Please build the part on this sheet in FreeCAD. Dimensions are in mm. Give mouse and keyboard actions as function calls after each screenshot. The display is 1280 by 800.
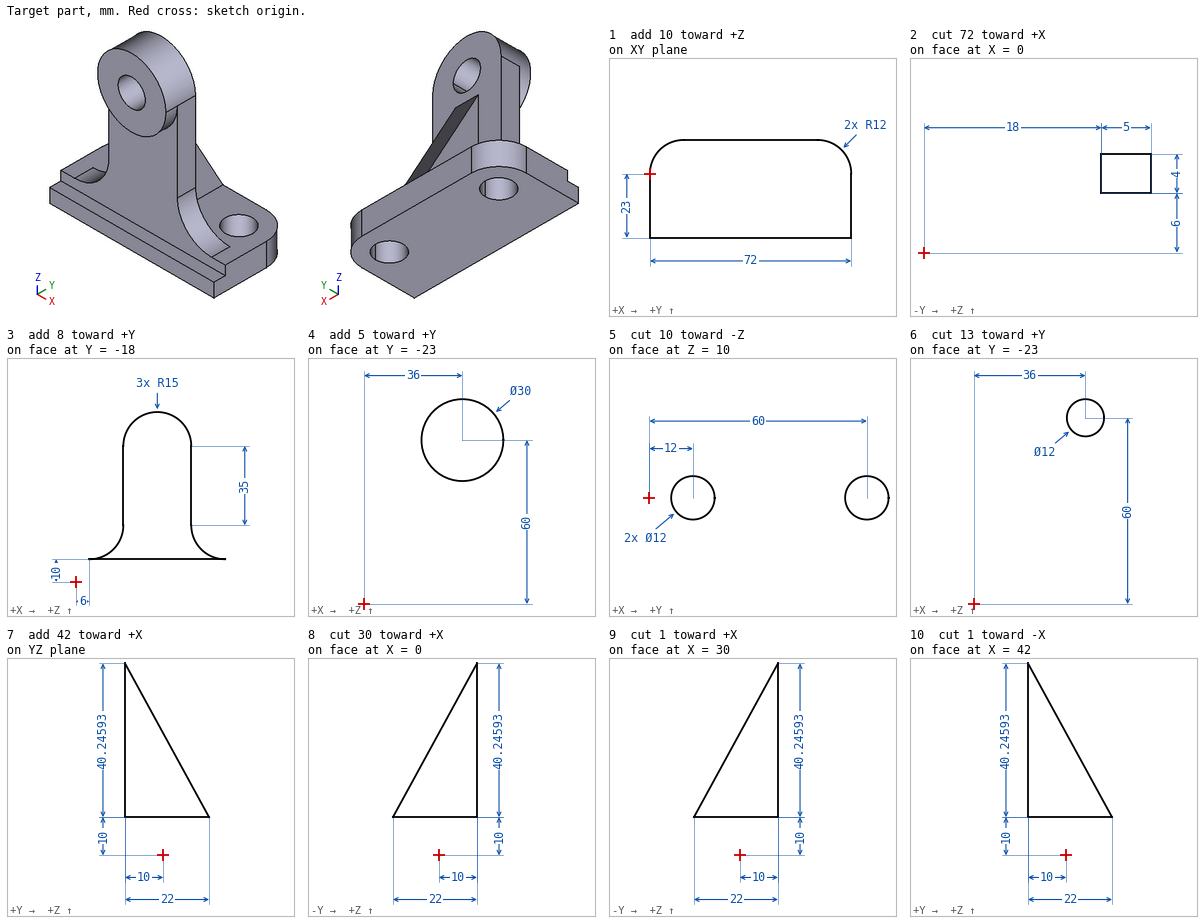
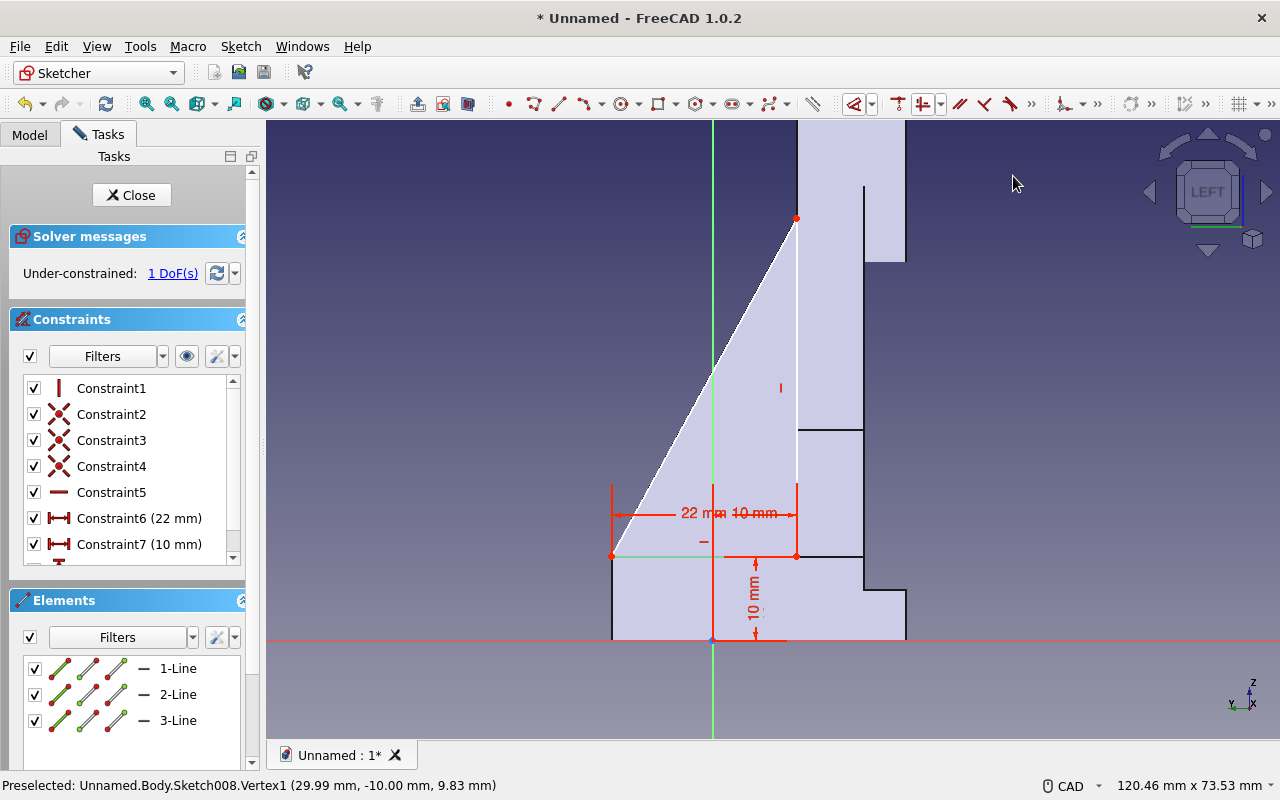
click(797, 455)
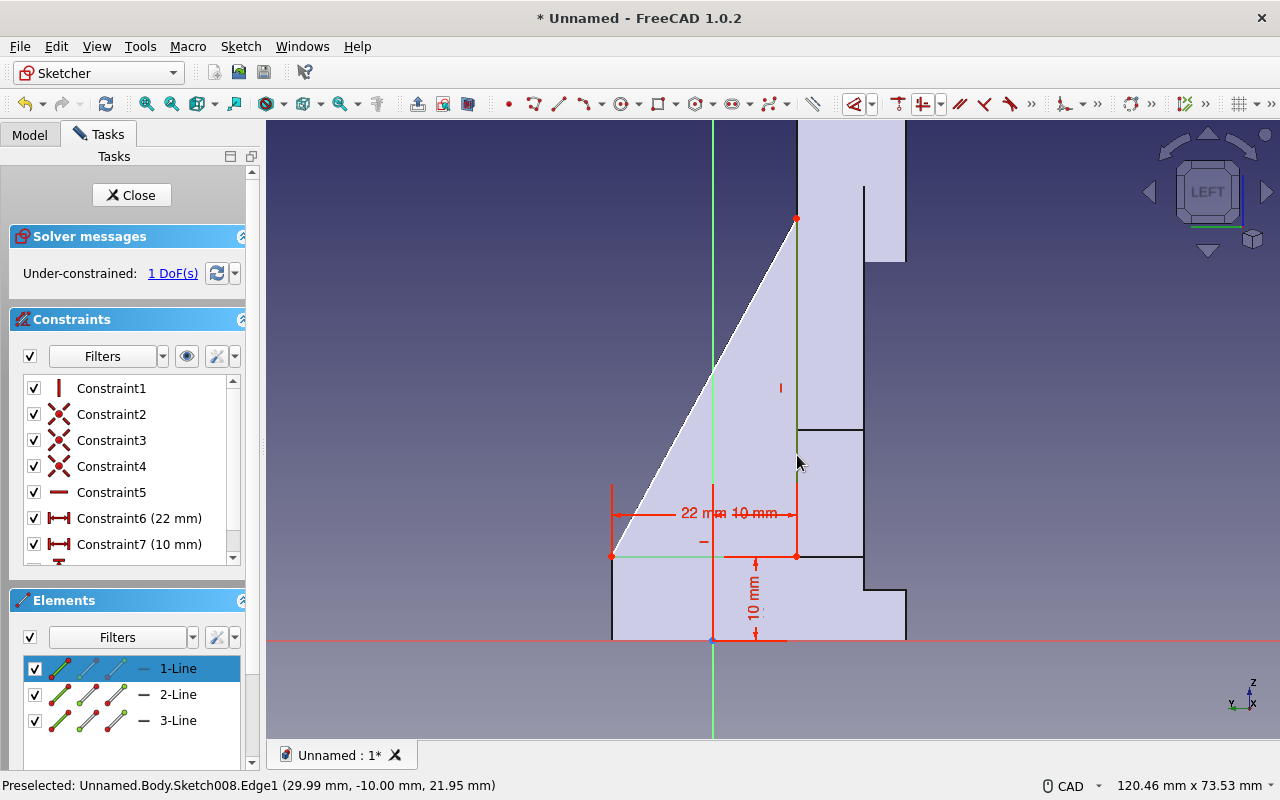
key(i)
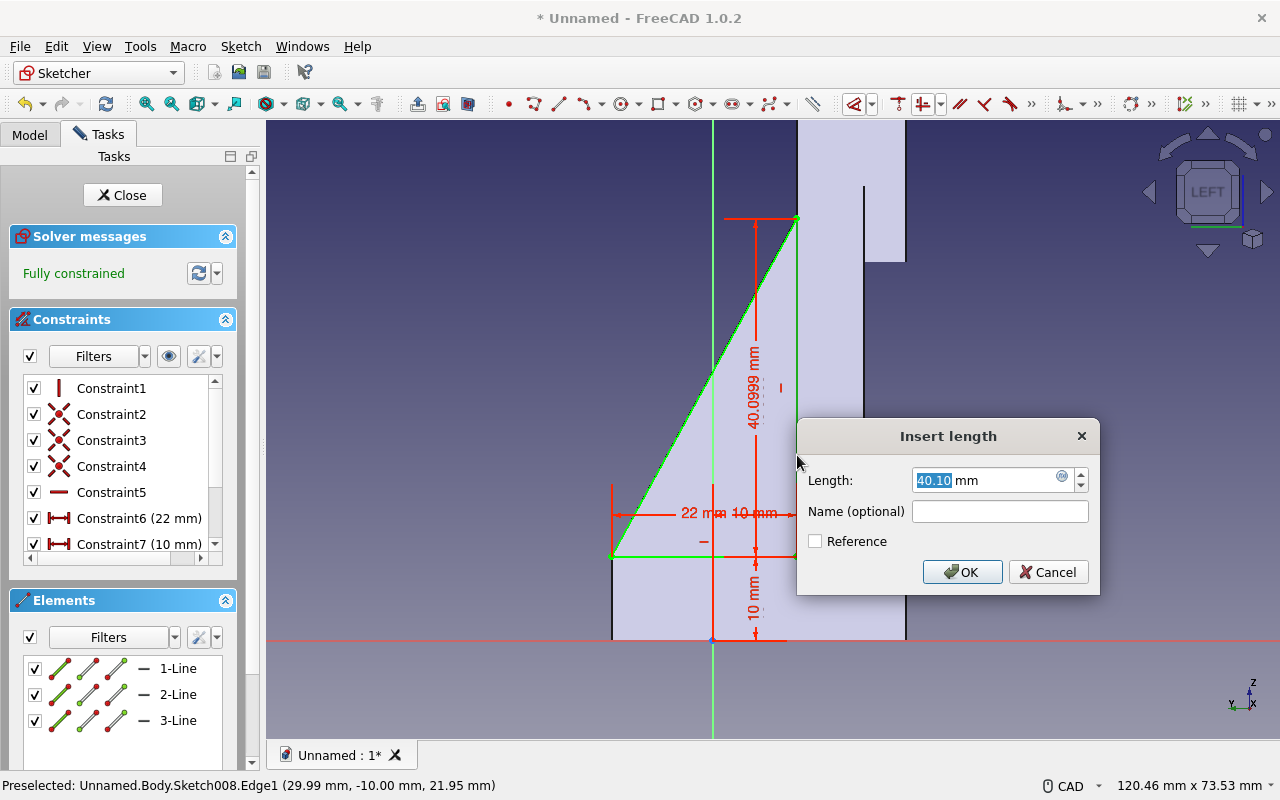
text(40.24593)
key(Return)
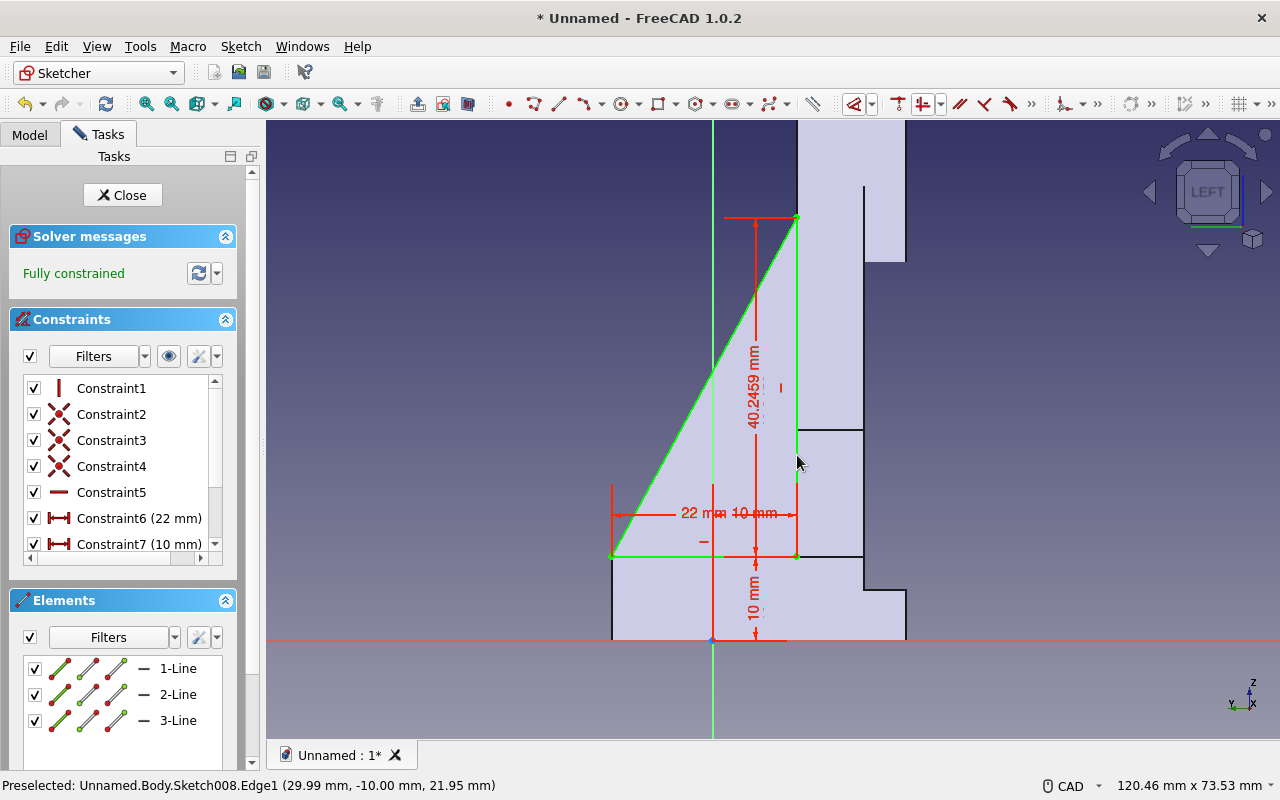
click(123, 195)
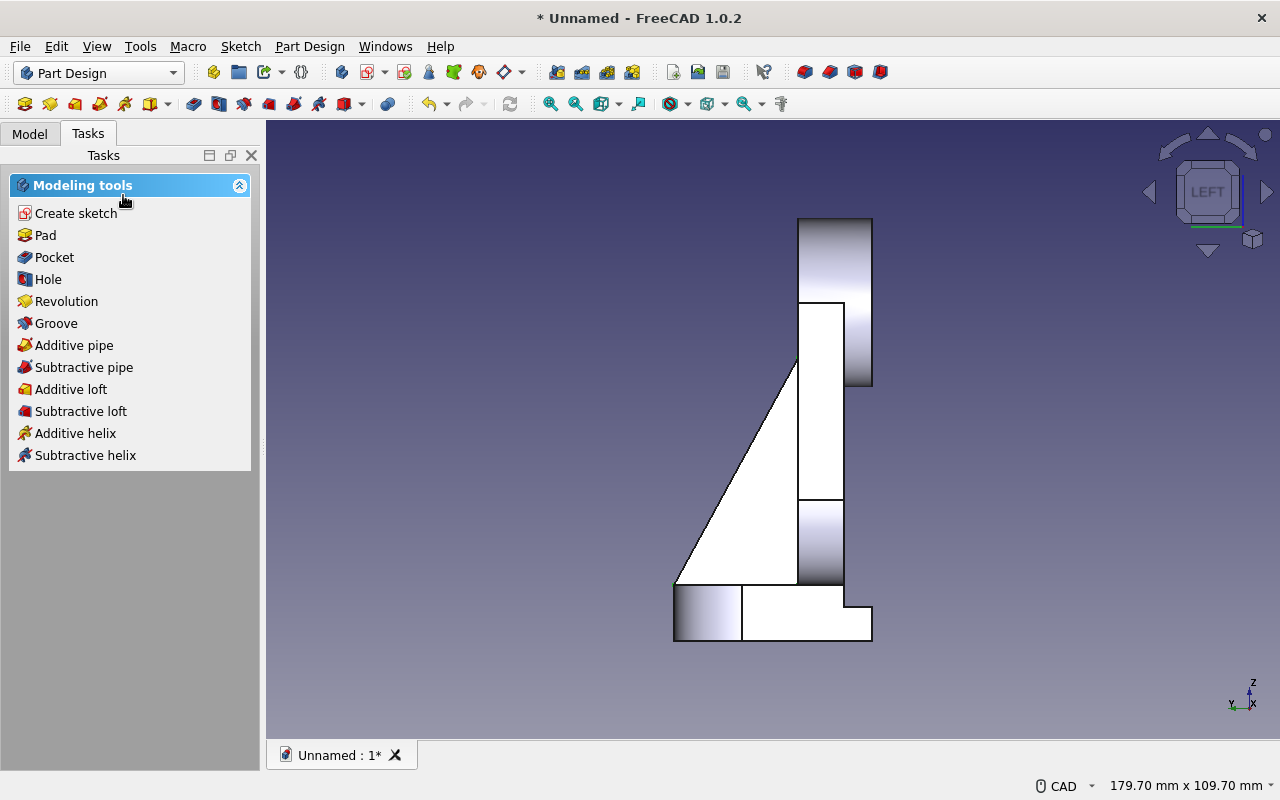
click(194, 104)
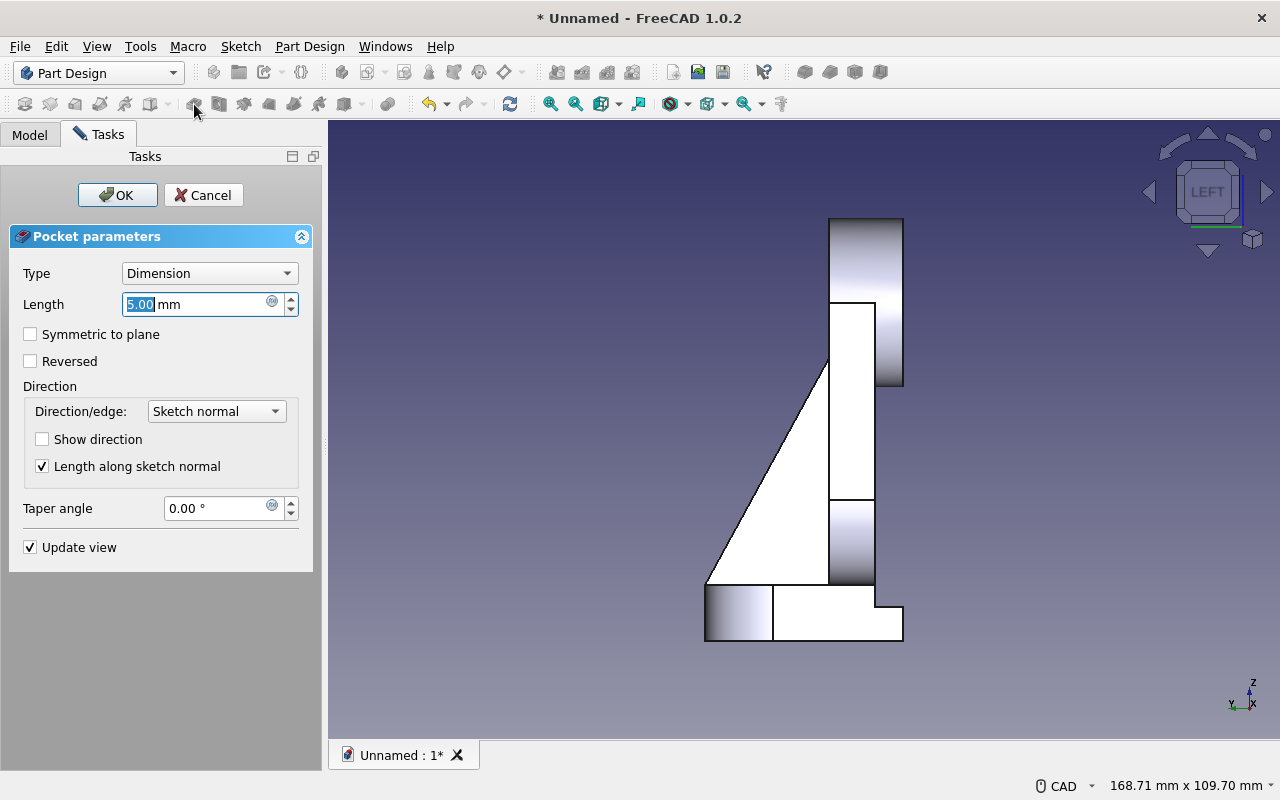
text(1)
key(Tab)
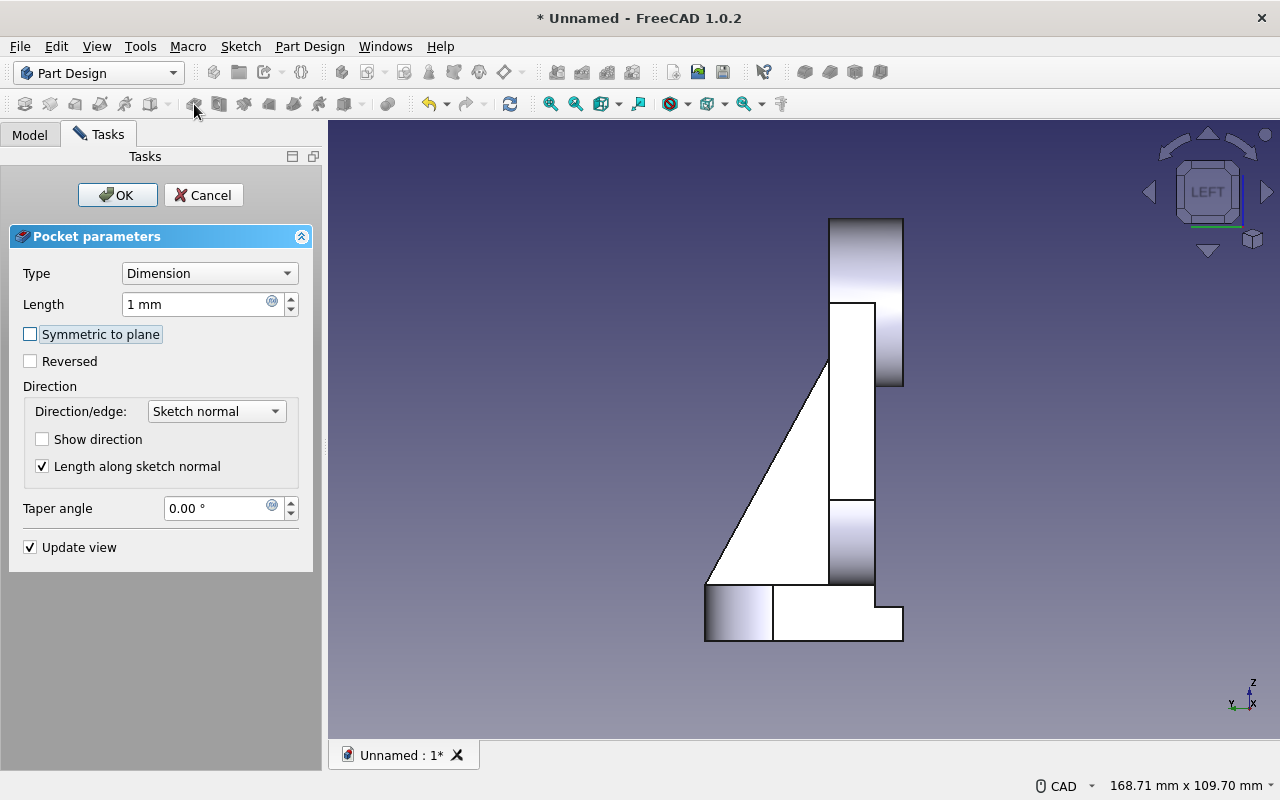
click(118, 195)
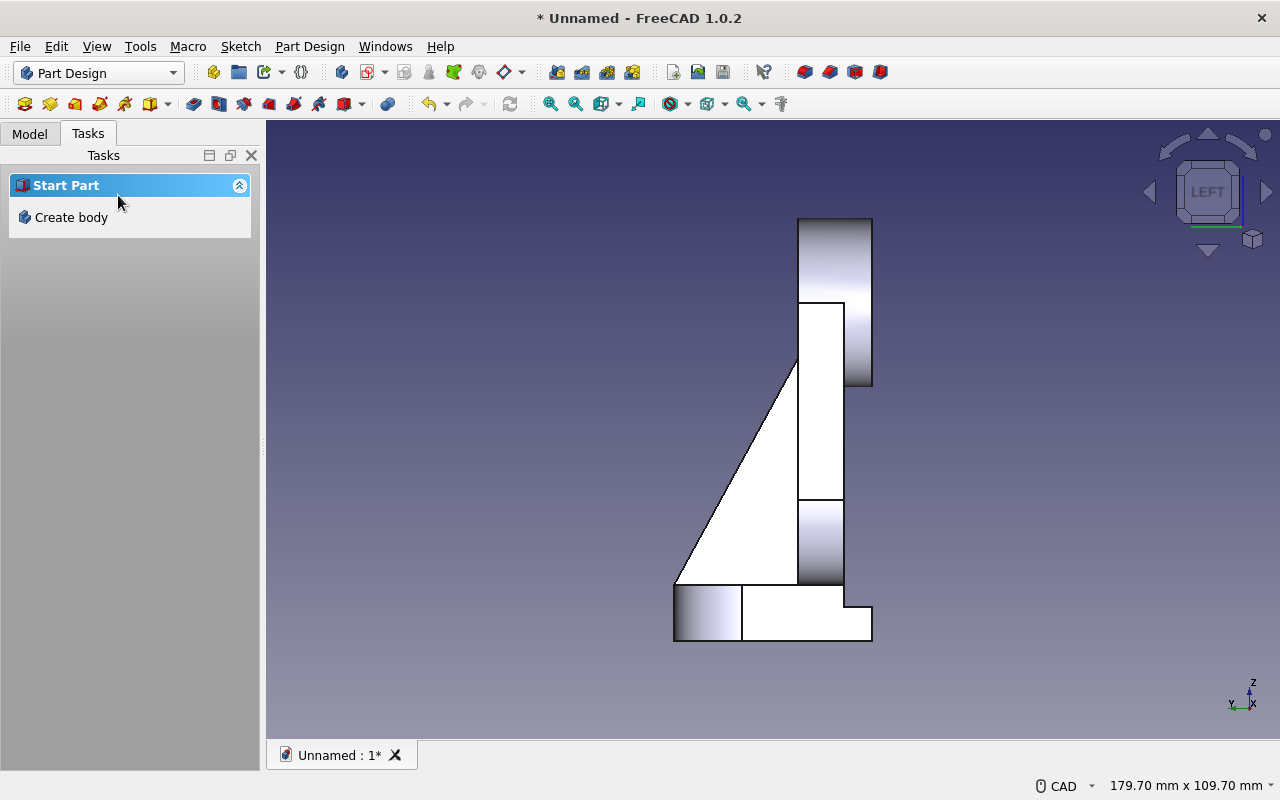
key(0)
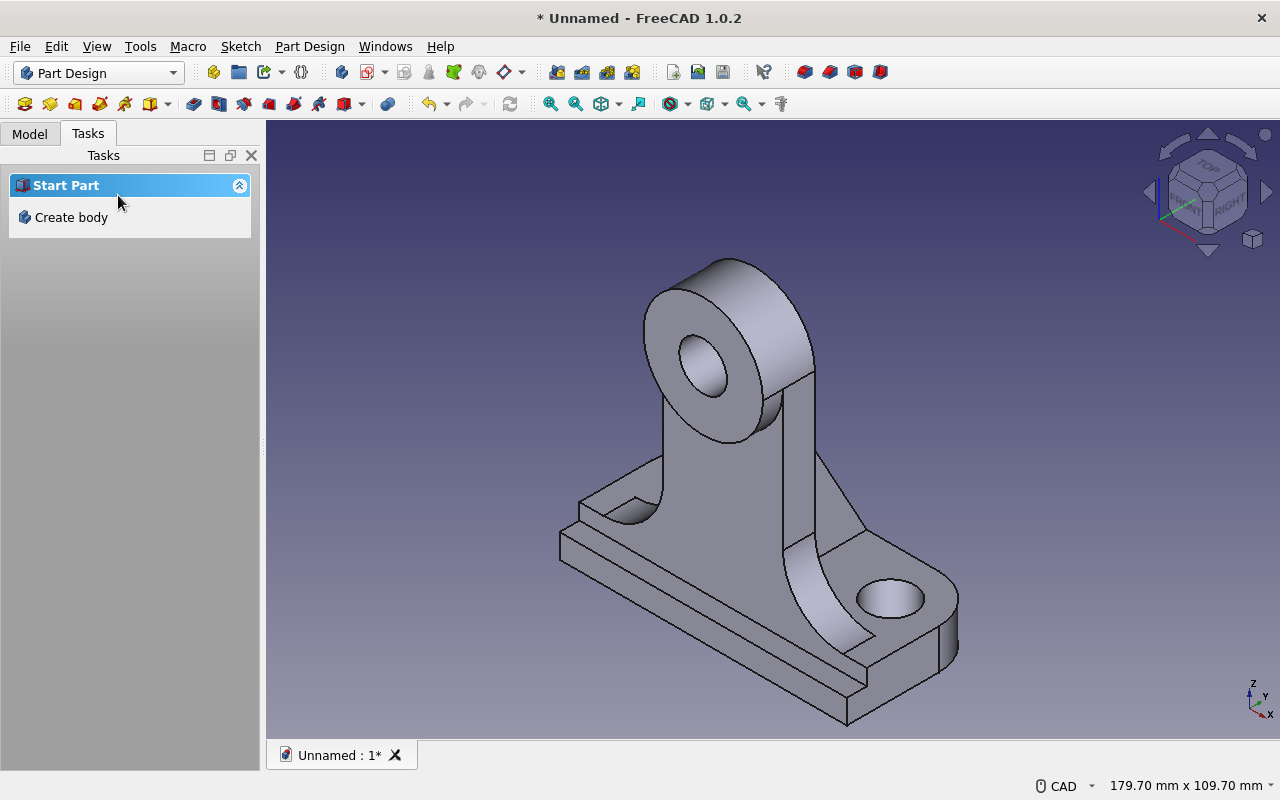
click(823, 514)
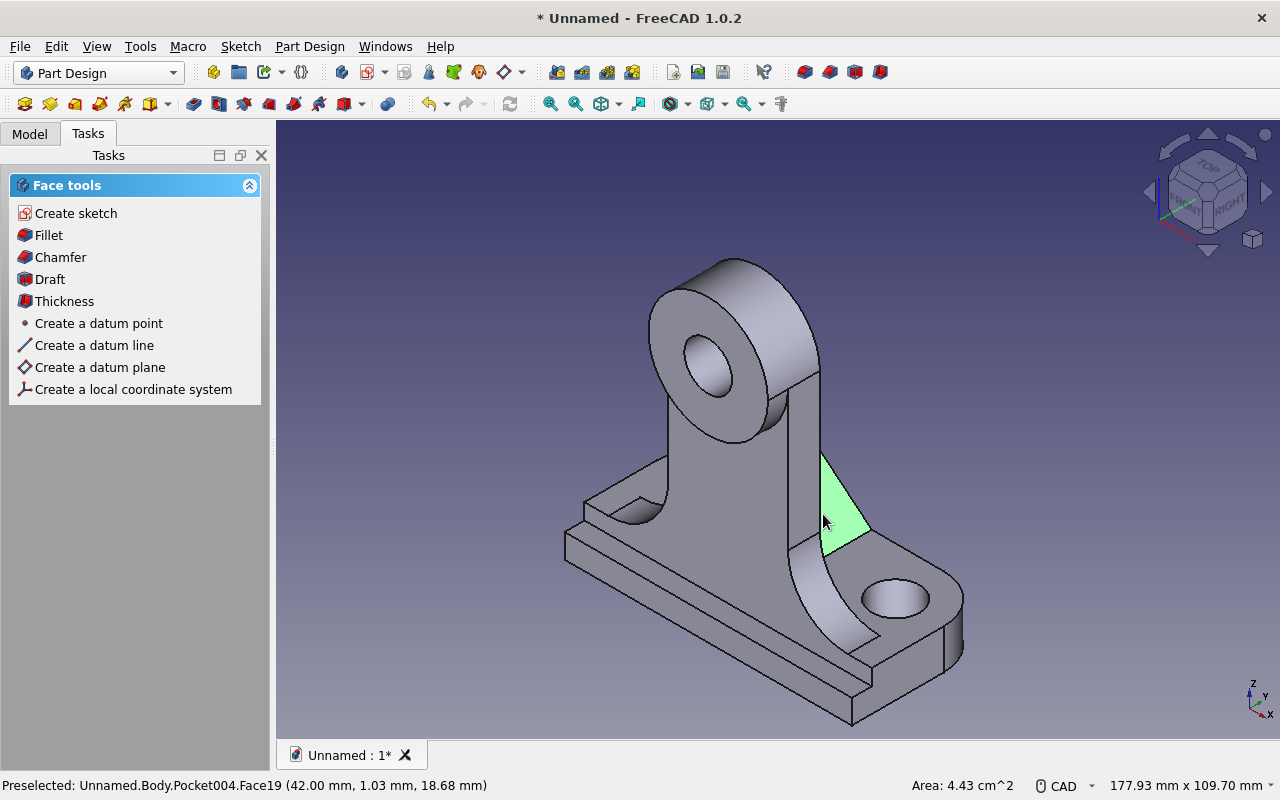
click(366, 72)